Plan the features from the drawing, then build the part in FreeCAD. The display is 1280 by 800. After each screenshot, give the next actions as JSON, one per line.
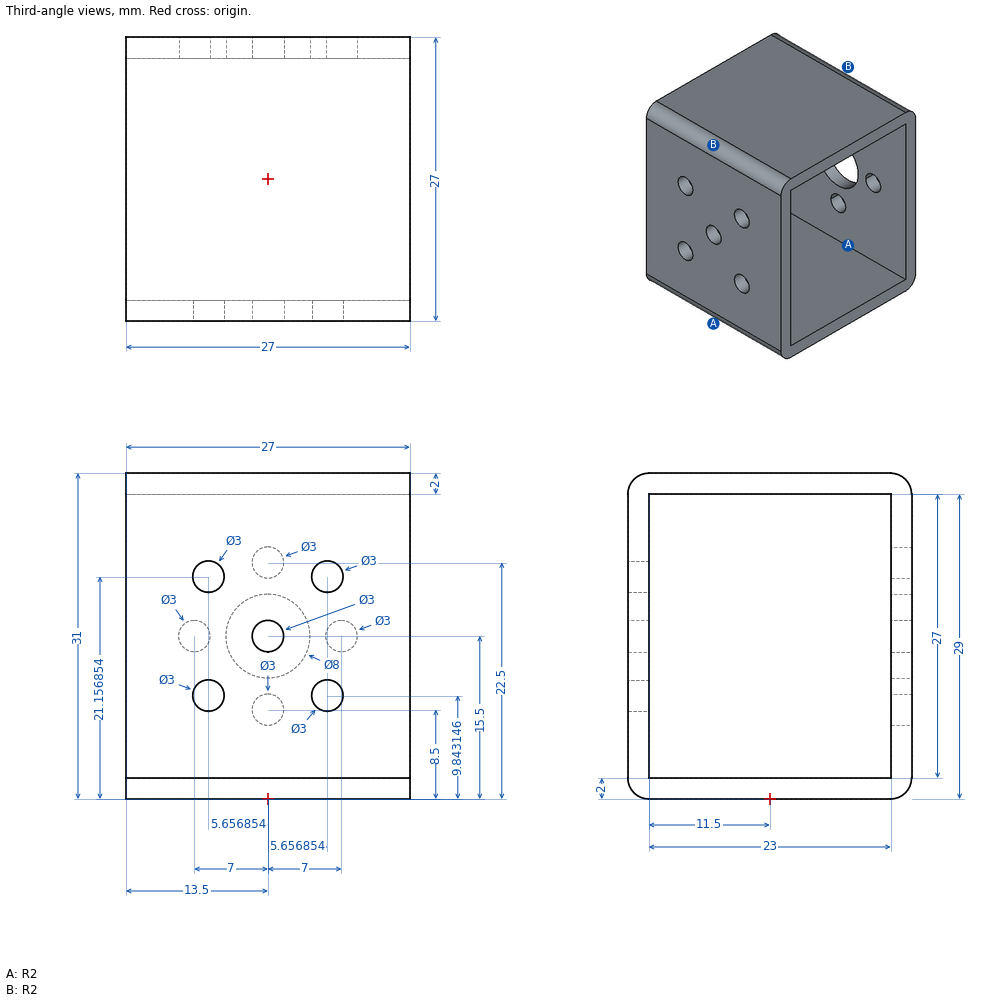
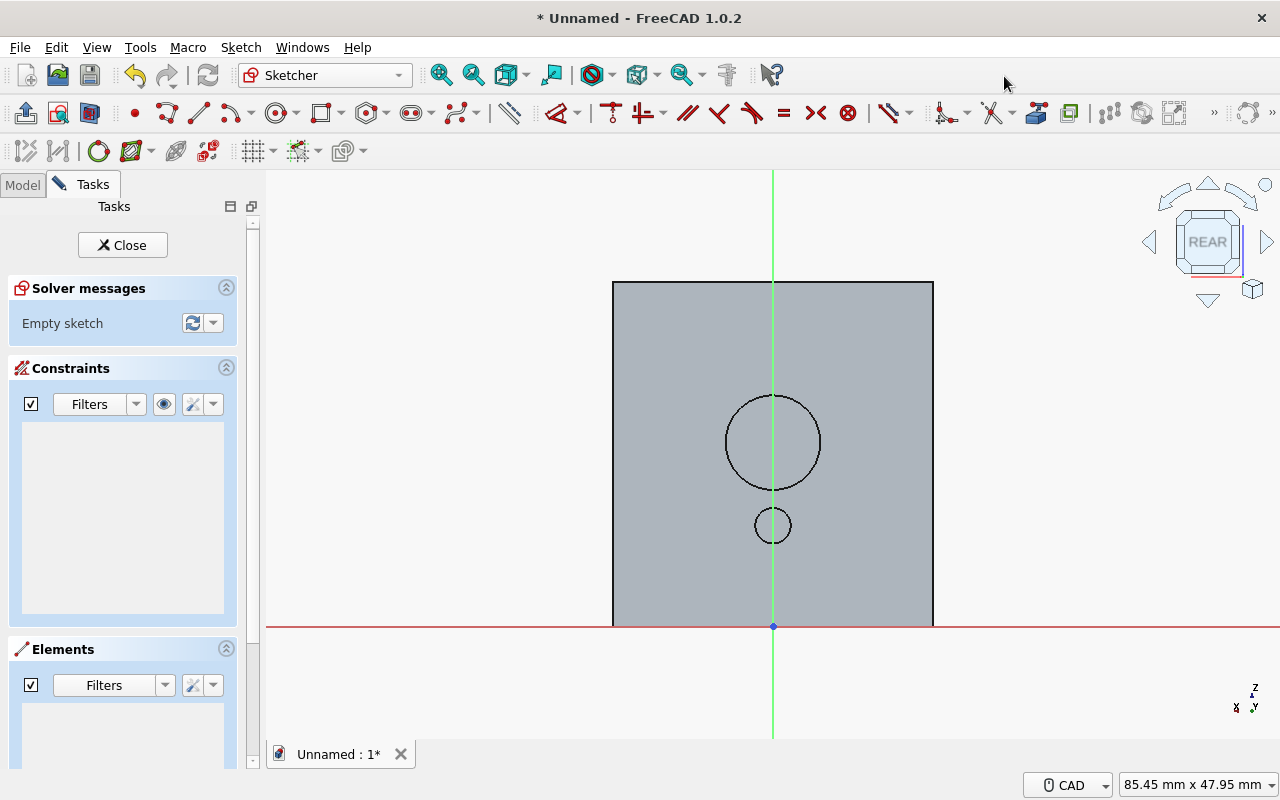
{"action": "scroll", "coordinate": [688, 441], "scroll_direction": "up", "scroll_amount": 12}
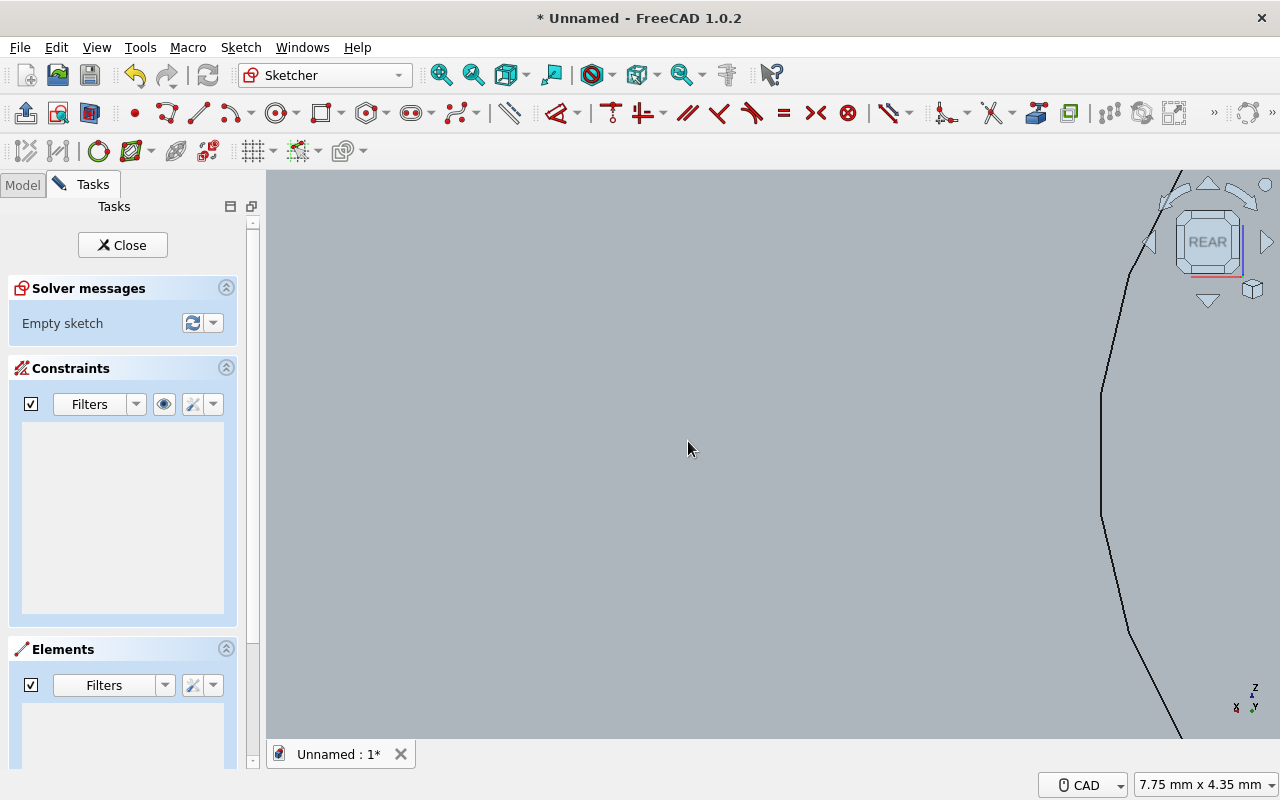
{"action": "left_click", "coordinate": [276, 114]}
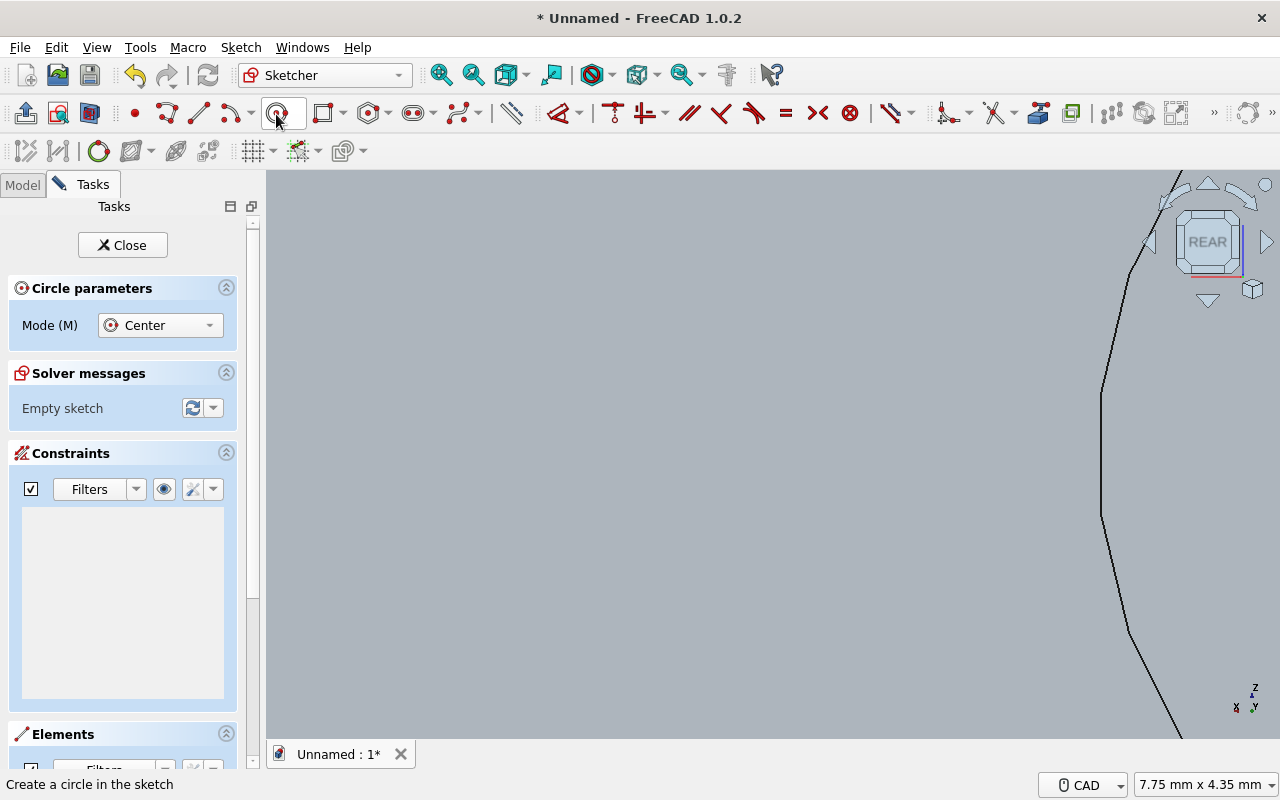
{"action": "left_click", "coordinate": [705, 454]}
{"action": "mouse_move", "coordinate": [844, 315]}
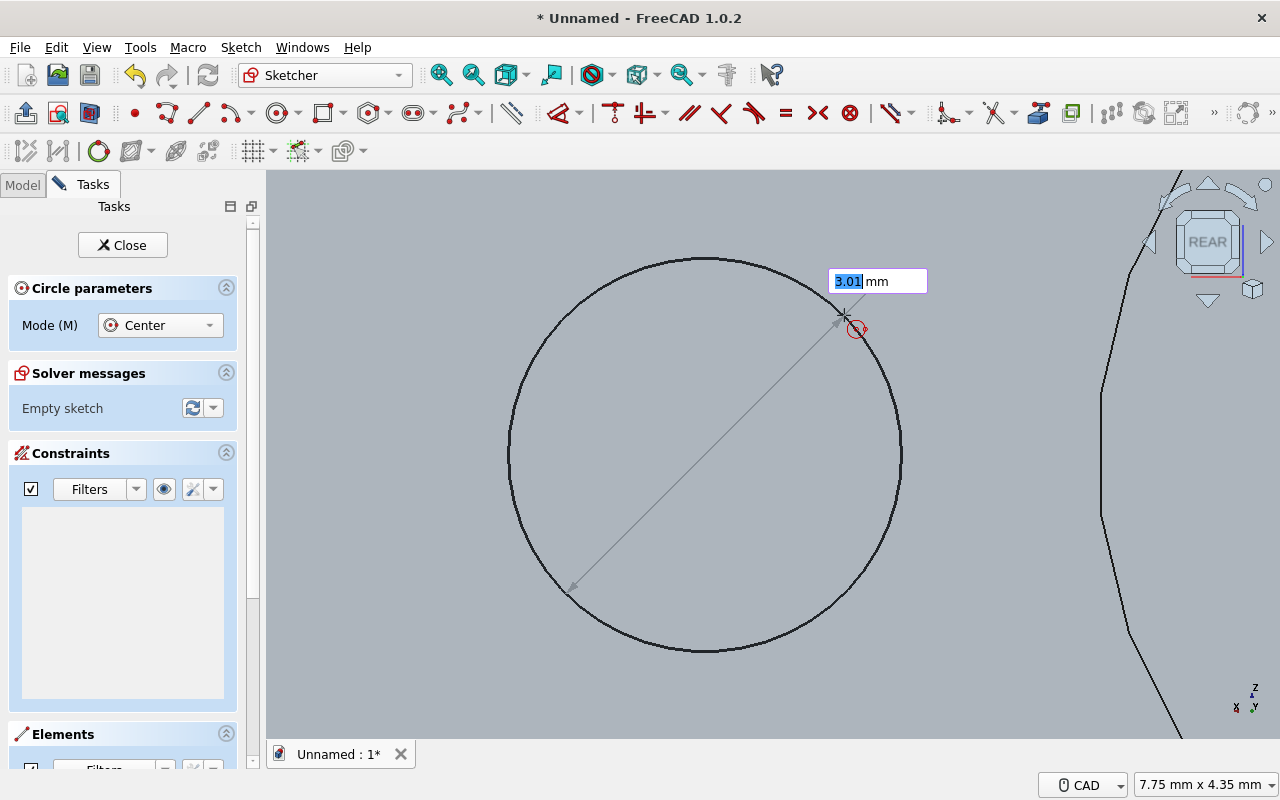
{"action": "type", "text": "3"}
{"action": "key", "text": "Return"}
{"action": "key", "text": "Escape"}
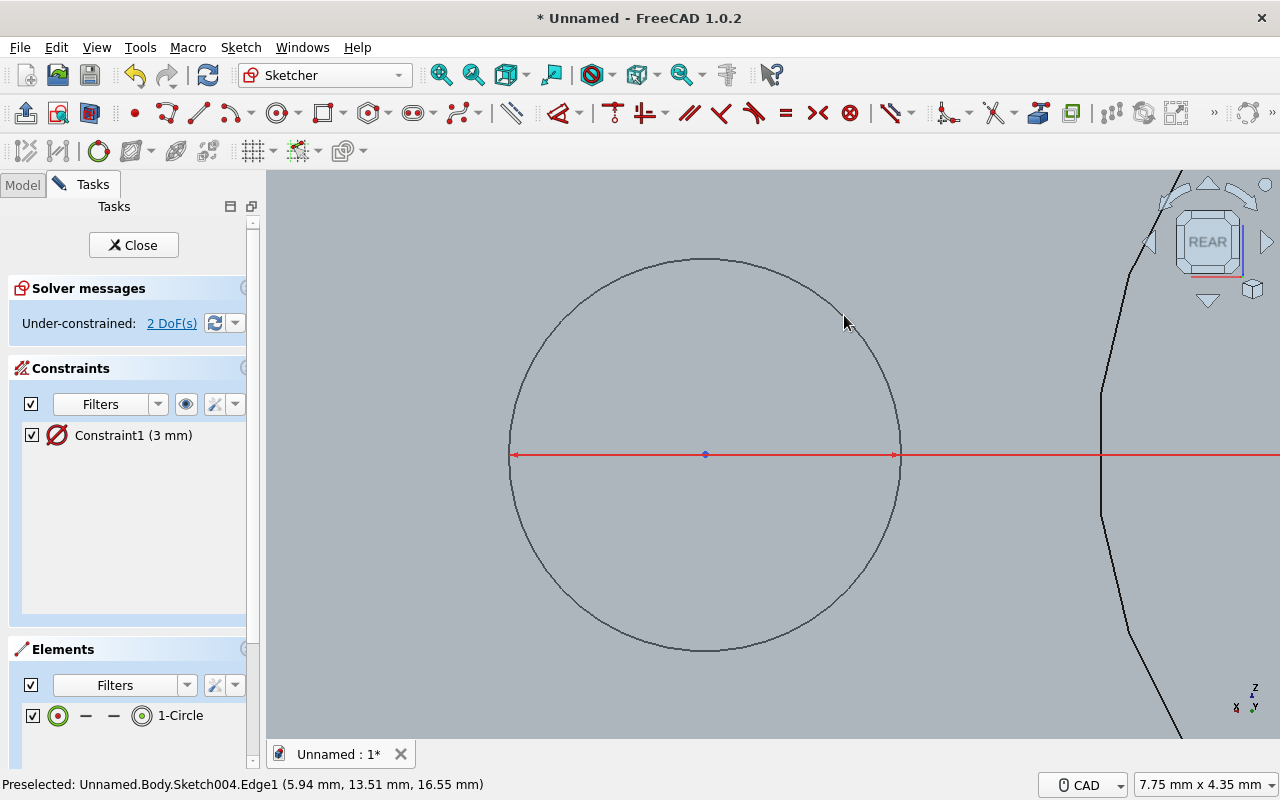
{"action": "left_click", "coordinate": [558, 114]}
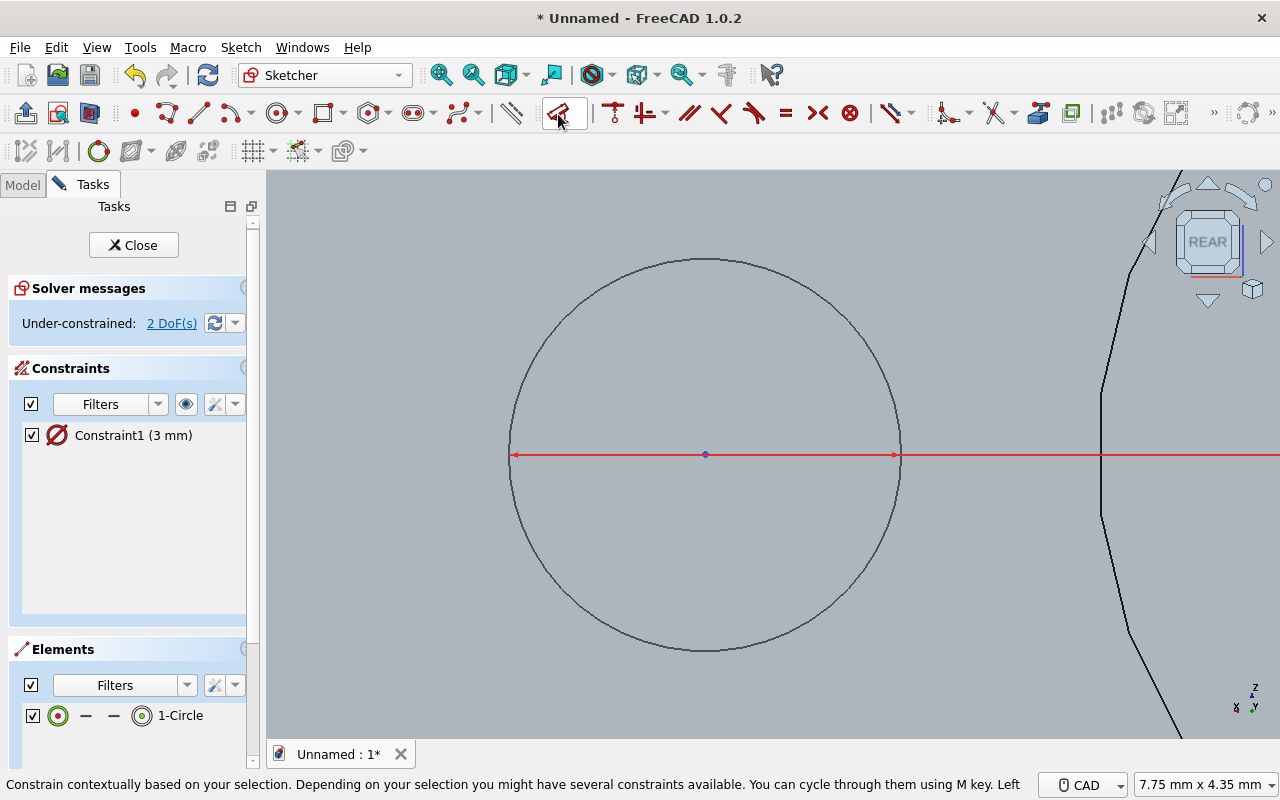
{"action": "left_click", "coordinate": [705, 455]}
{"action": "left_click", "coordinate": [816, 421]}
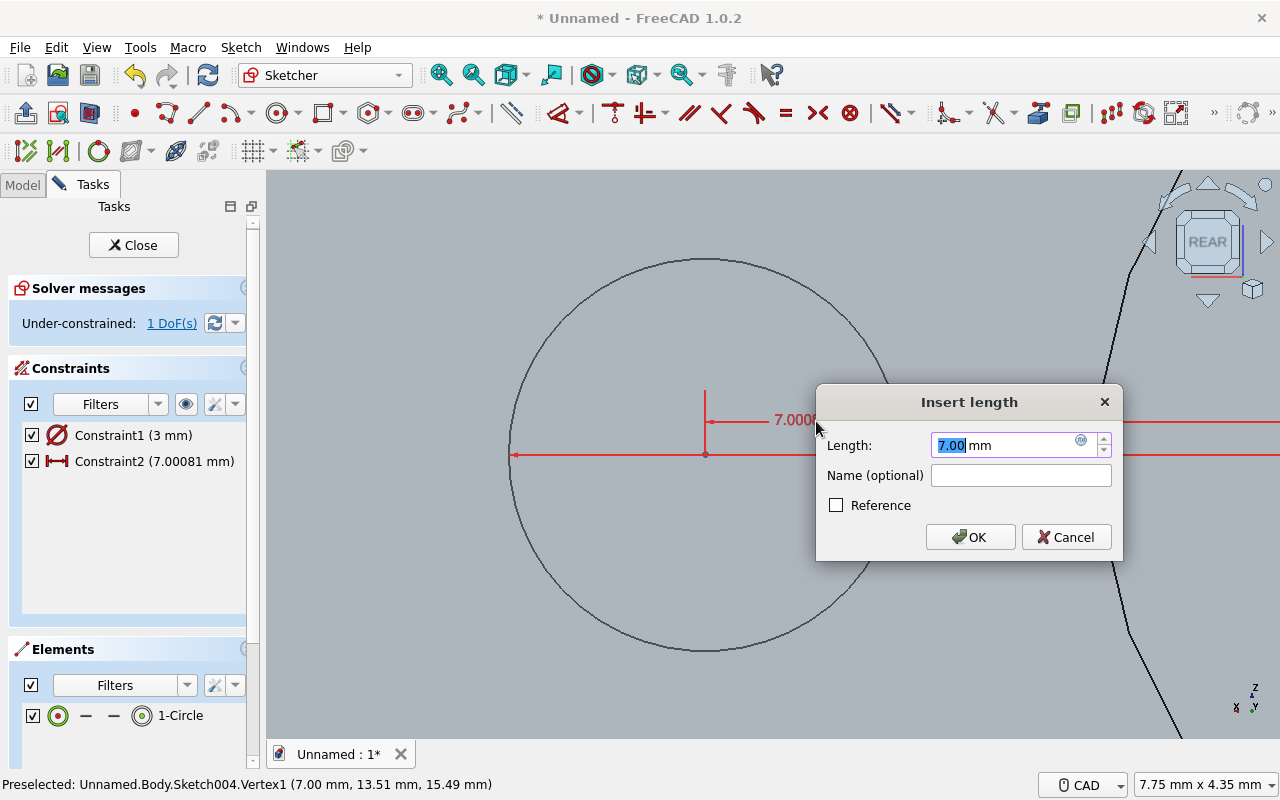
{"action": "type", "text": "7"}
{"action": "key", "text": "Return"}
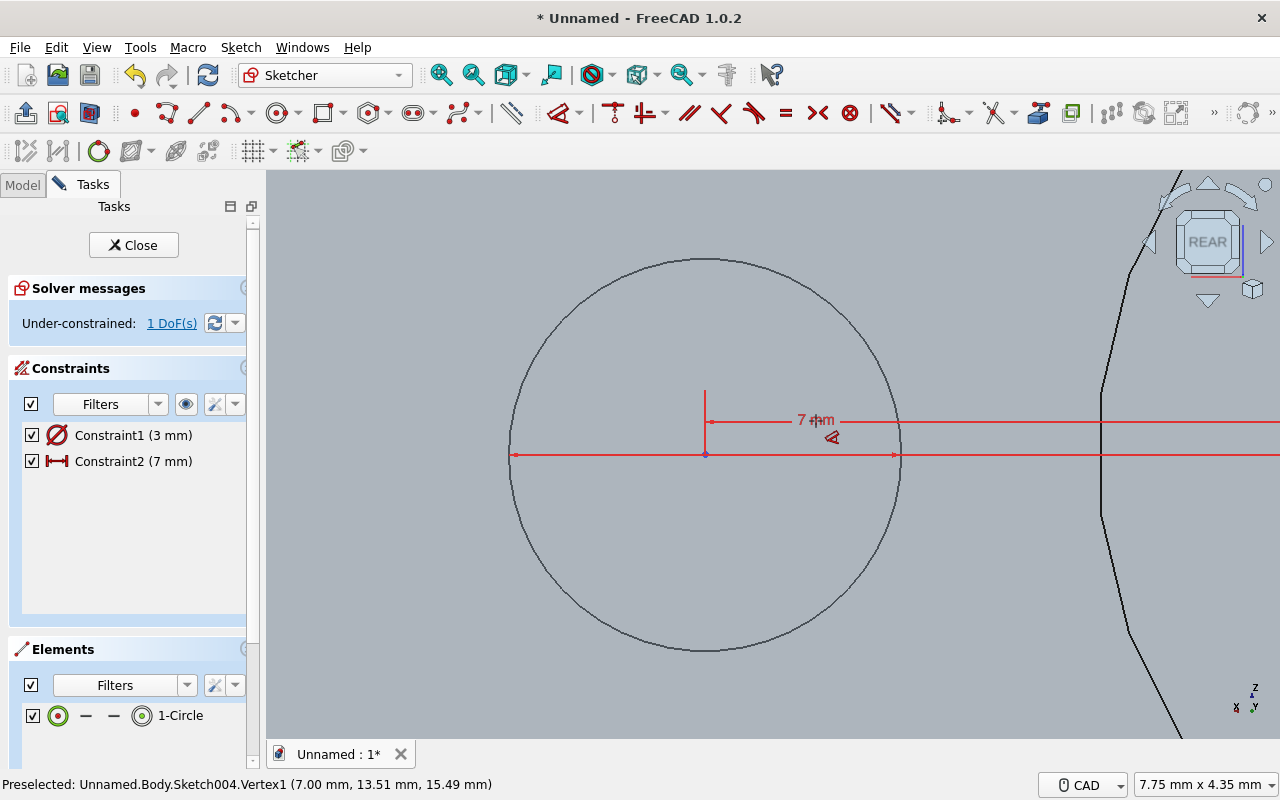
{"action": "left_click", "coordinate": [705, 455]}
{"action": "left_click", "coordinate": [671, 583]}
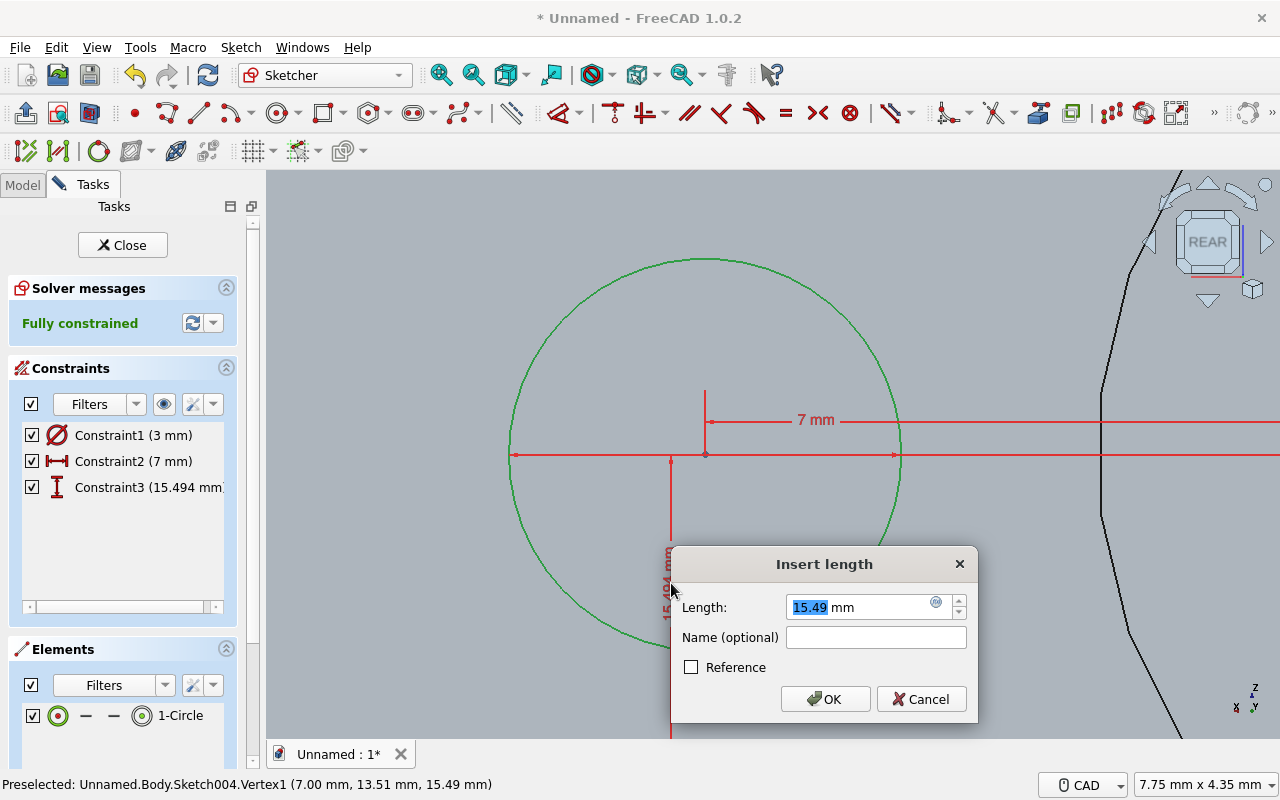
{"action": "type", "text": "15.5"}
{"action": "key", "text": "Return"}
{"action": "key", "text": "Escape"}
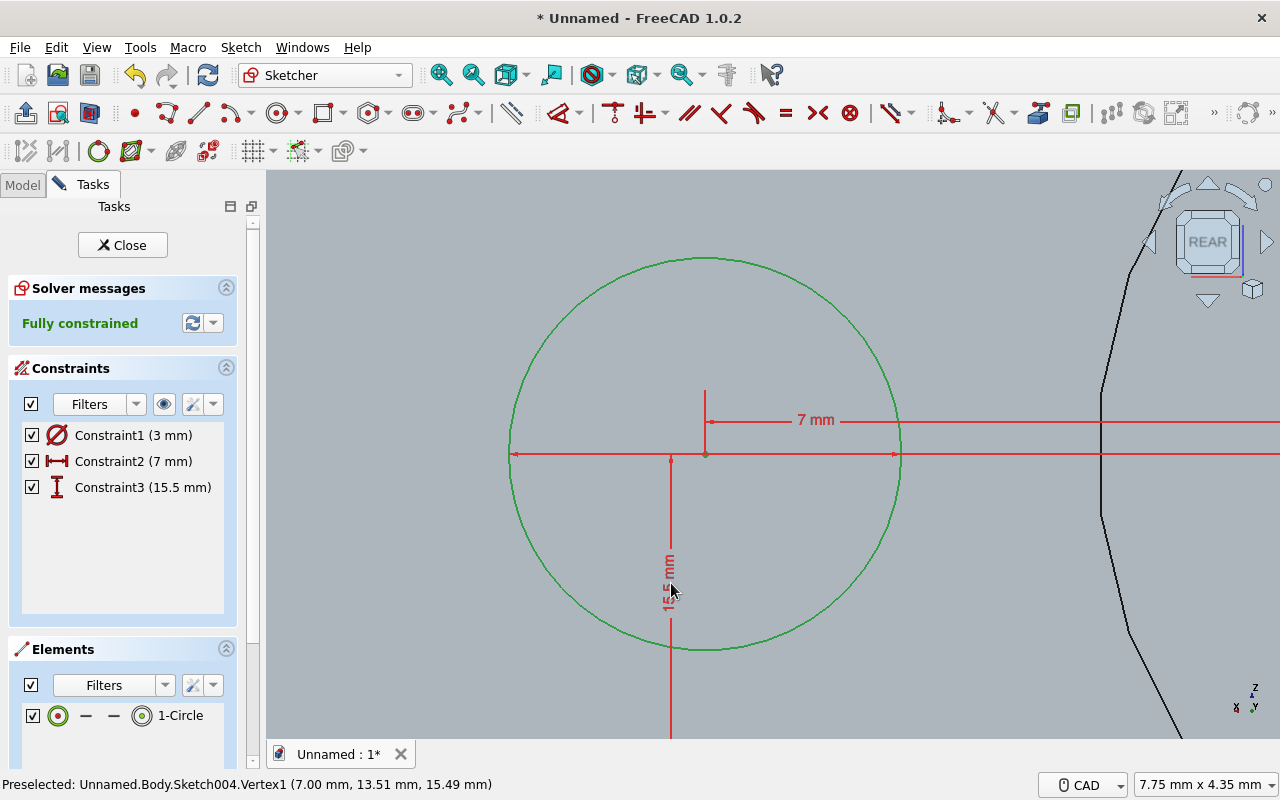
{"action": "left_click", "coordinate": [123, 245]}